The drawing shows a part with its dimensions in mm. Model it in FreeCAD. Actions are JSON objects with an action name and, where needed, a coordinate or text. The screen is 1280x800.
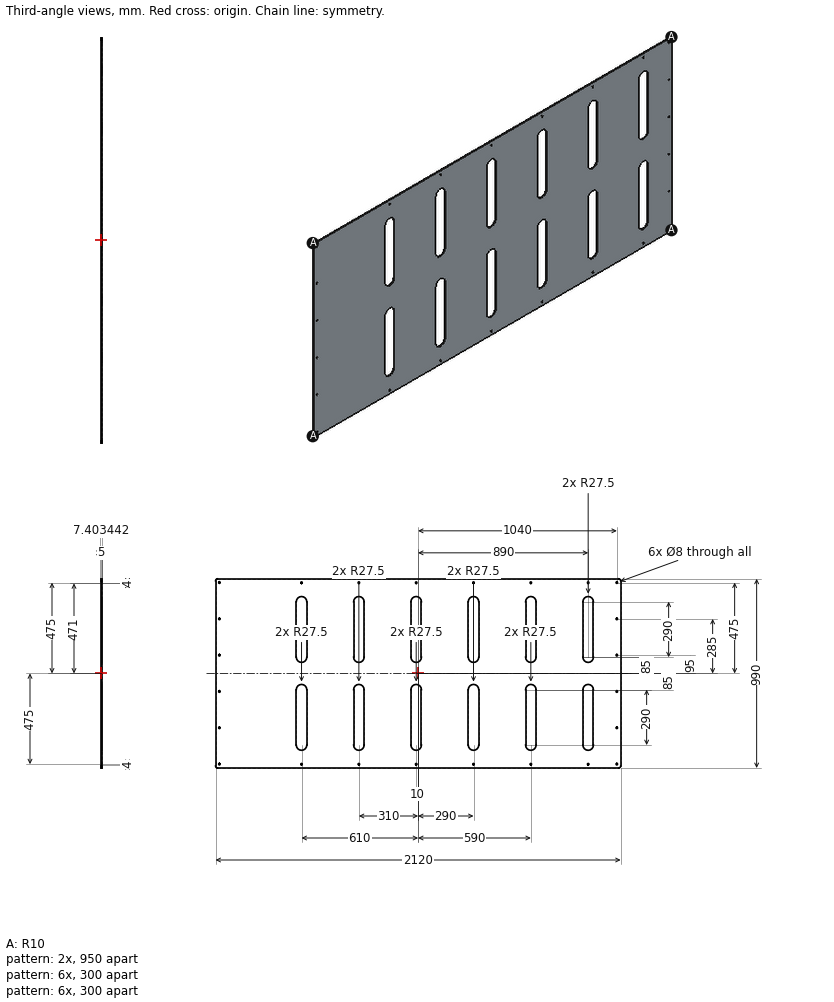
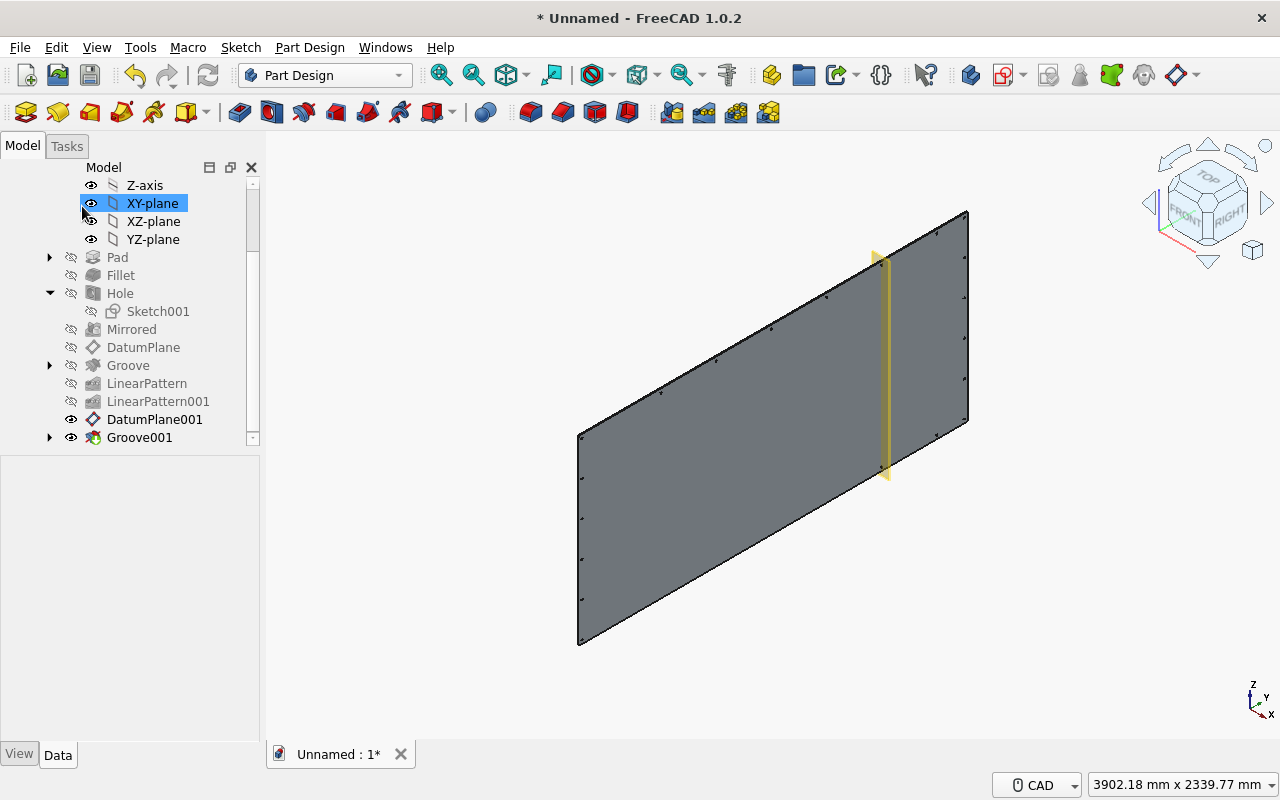
{"action": "left_click", "coordinate": [116, 419]}
{"action": "key", "text": "space"}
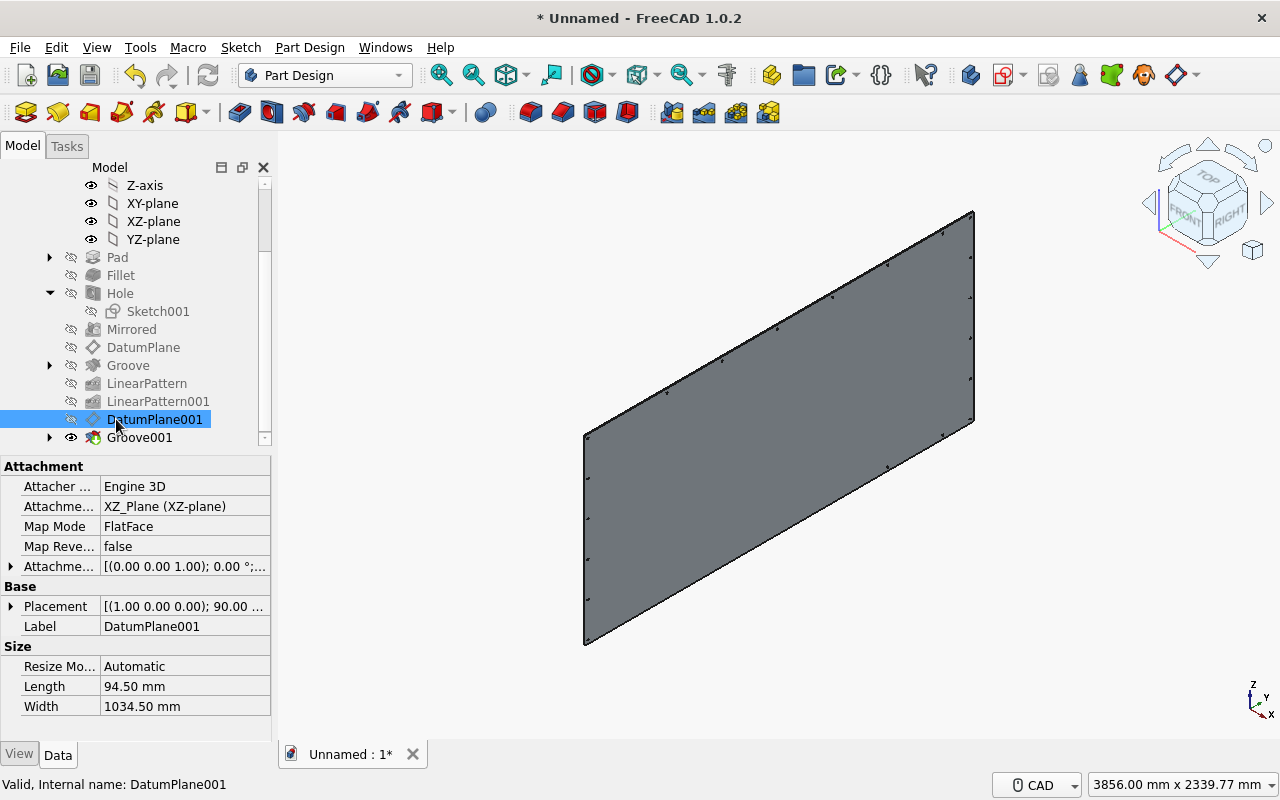
{"action": "scroll", "coordinate": [160, 307], "scroll_direction": "down", "scroll_amount": 3}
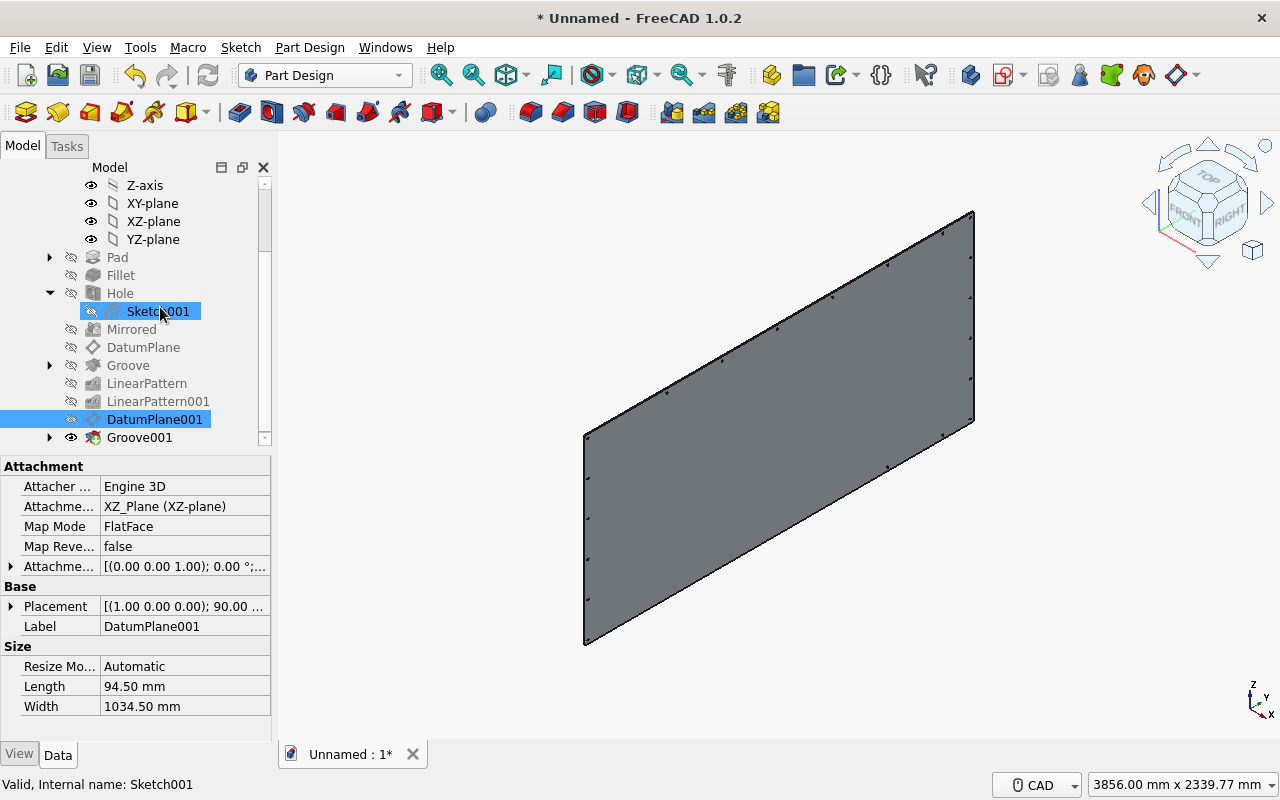
{"action": "scroll", "coordinate": [160, 307], "scroll_direction": "up", "scroll_amount": 15}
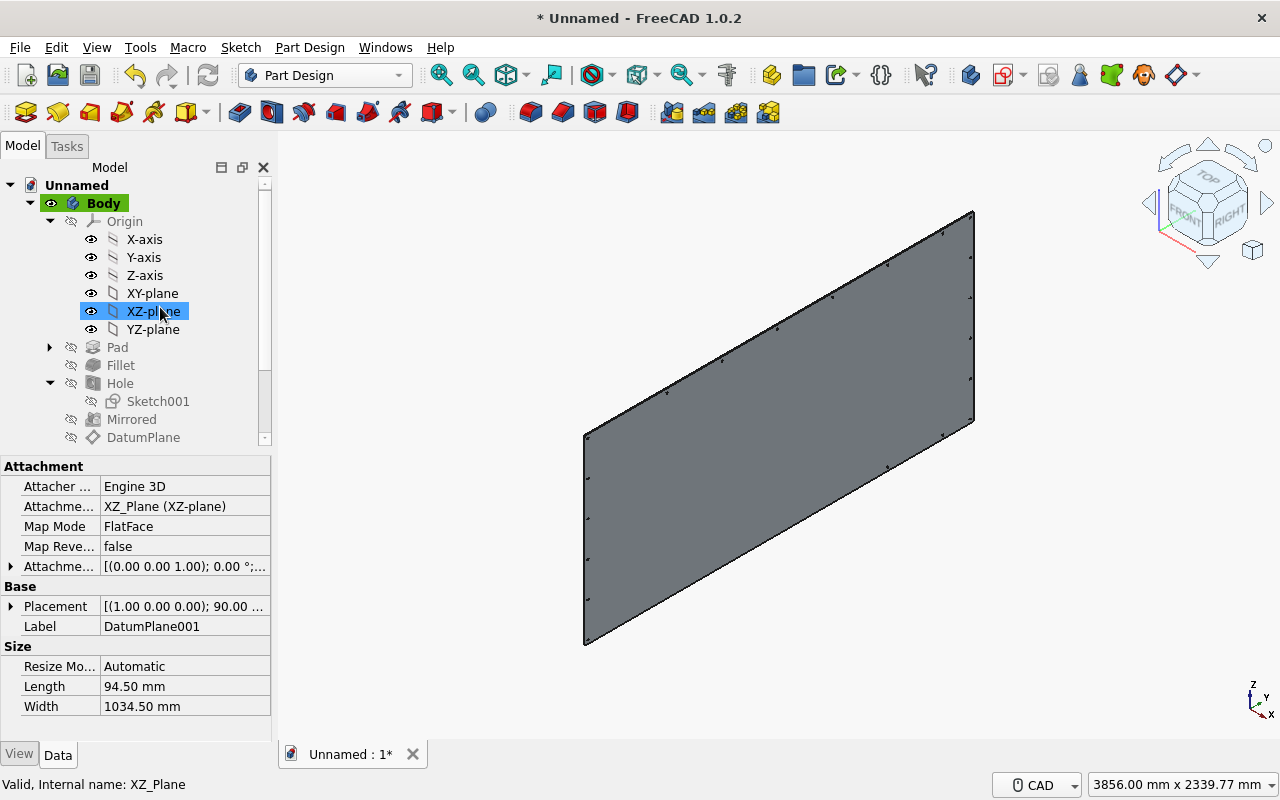
{"action": "left_click", "coordinate": [136, 311]}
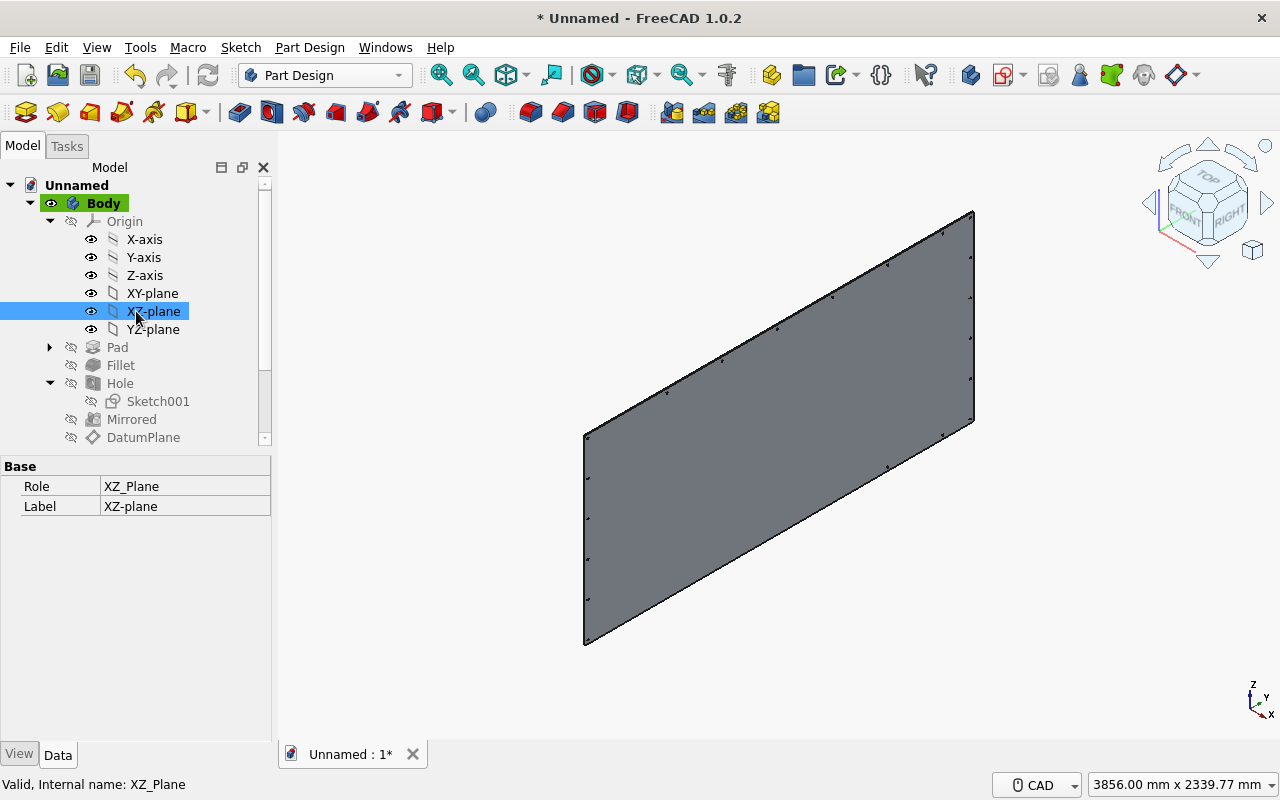
{"action": "left_click", "coordinate": [1176, 76]}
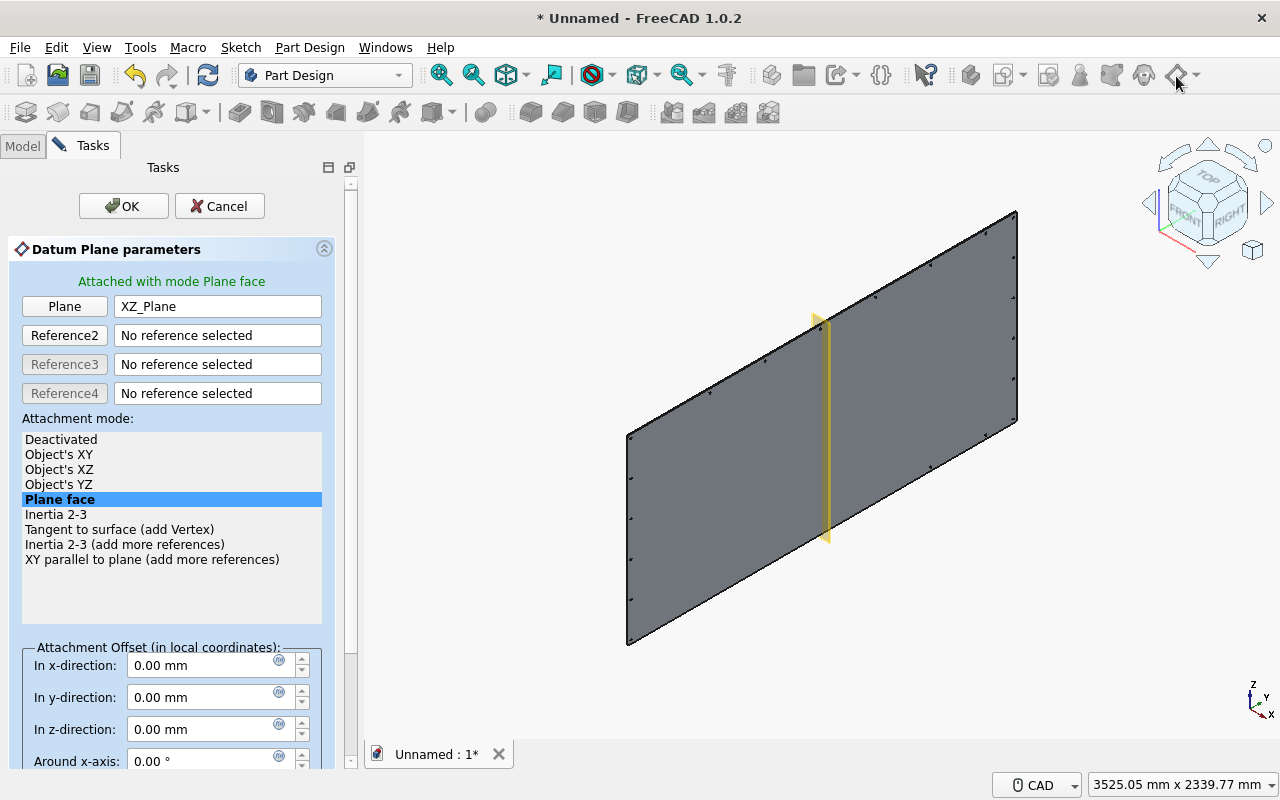
{"action": "triple_click", "coordinate": [210, 729]}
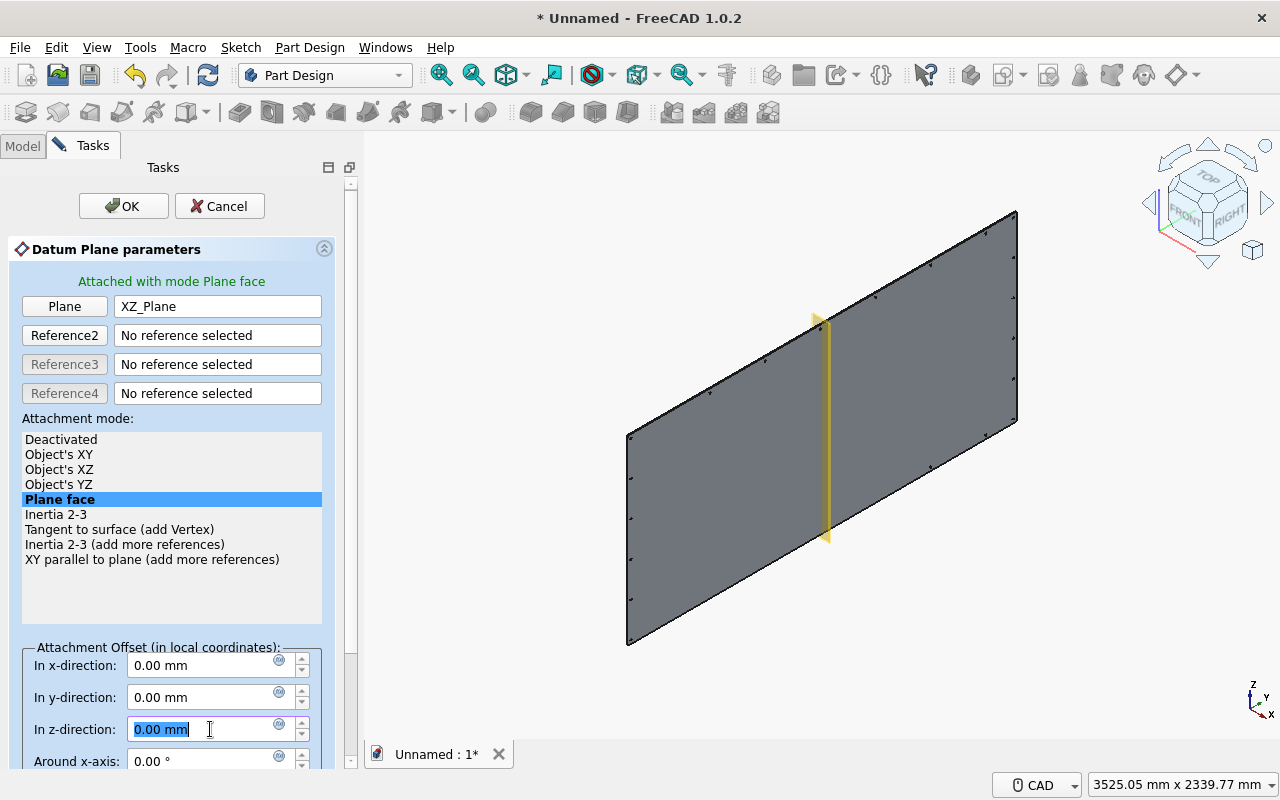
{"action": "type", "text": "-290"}
{"action": "key", "text": "Tab"}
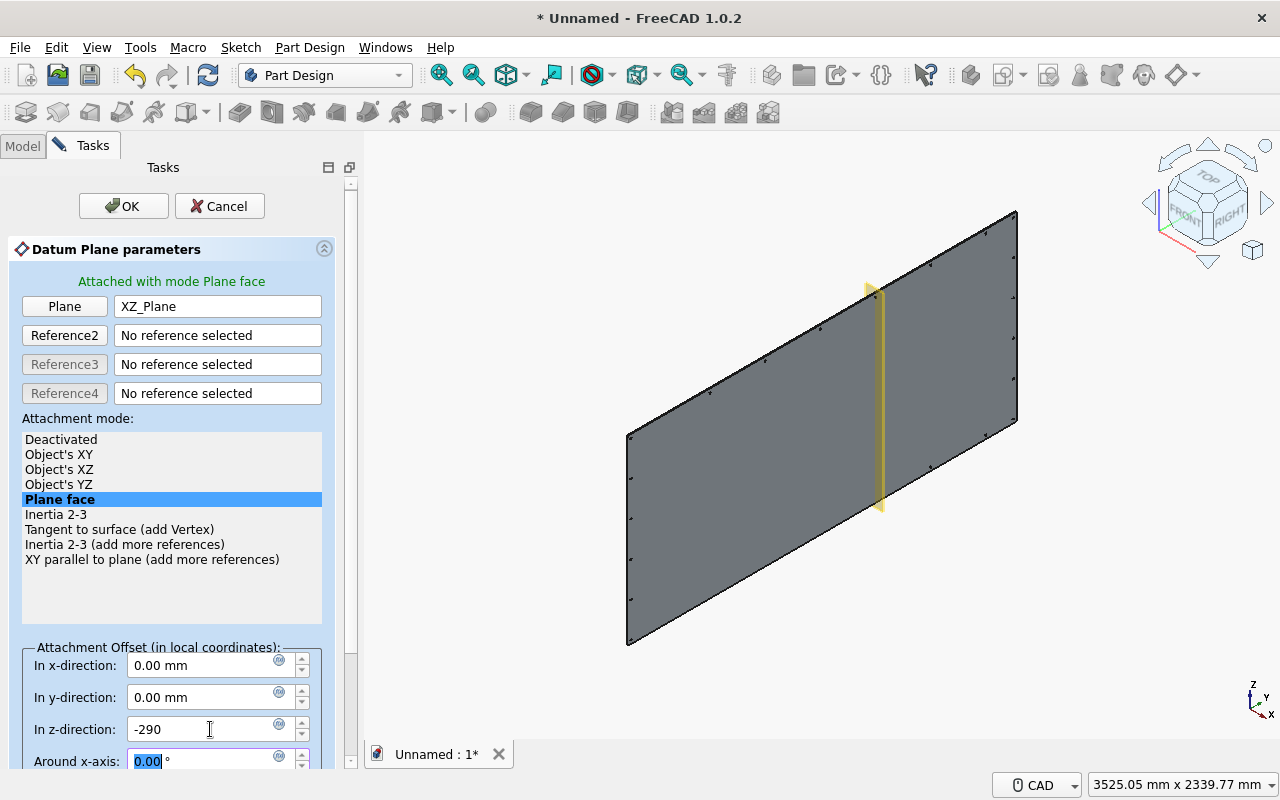
{"action": "left_click", "coordinate": [124, 206]}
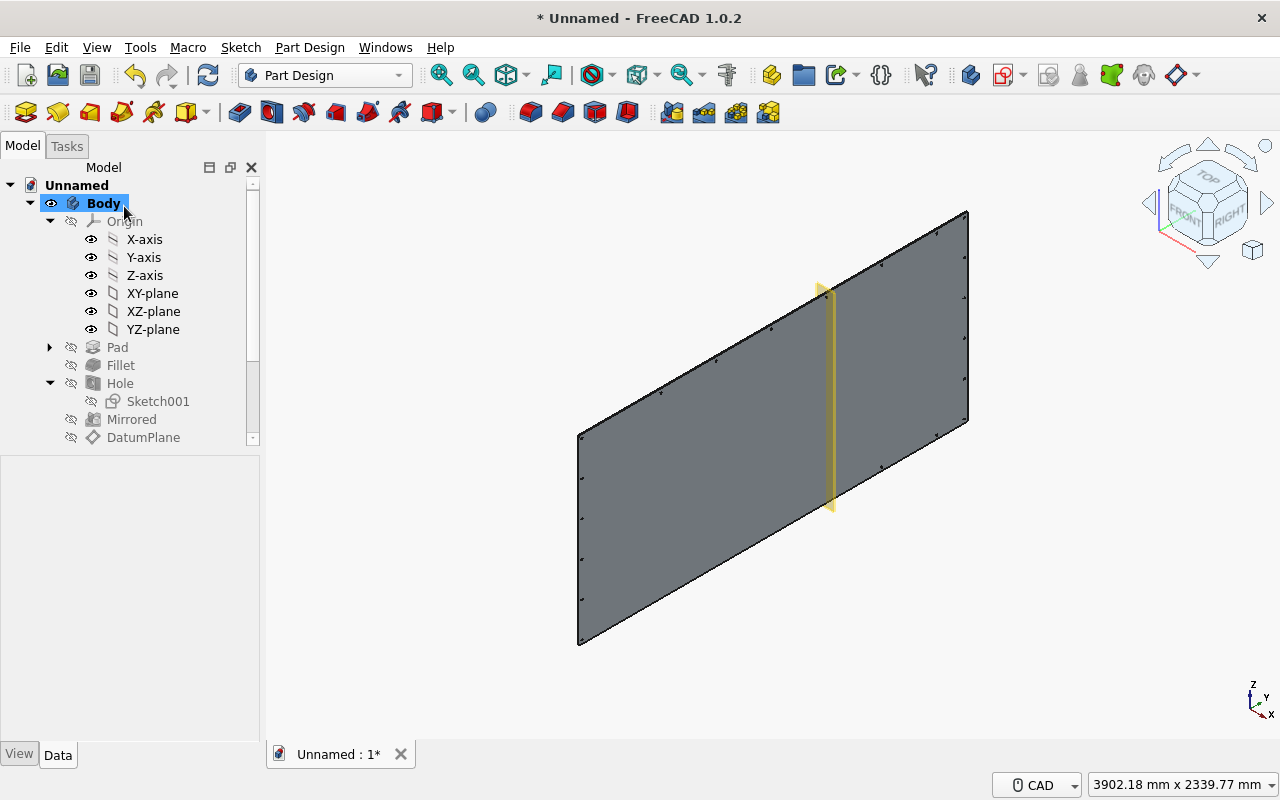
{"action": "scroll", "coordinate": [100, 307], "scroll_direction": "down", "scroll_amount": 3}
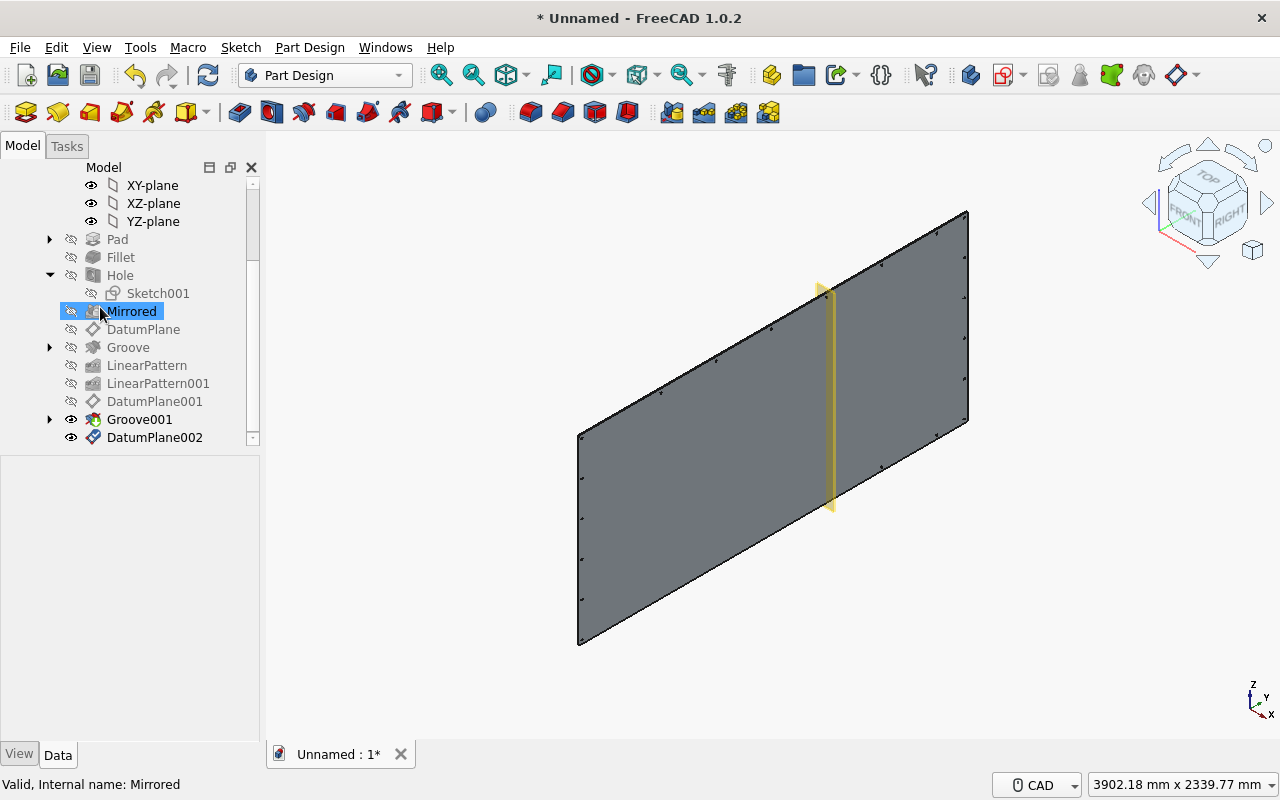
{"action": "left_click", "coordinate": [116, 437]}